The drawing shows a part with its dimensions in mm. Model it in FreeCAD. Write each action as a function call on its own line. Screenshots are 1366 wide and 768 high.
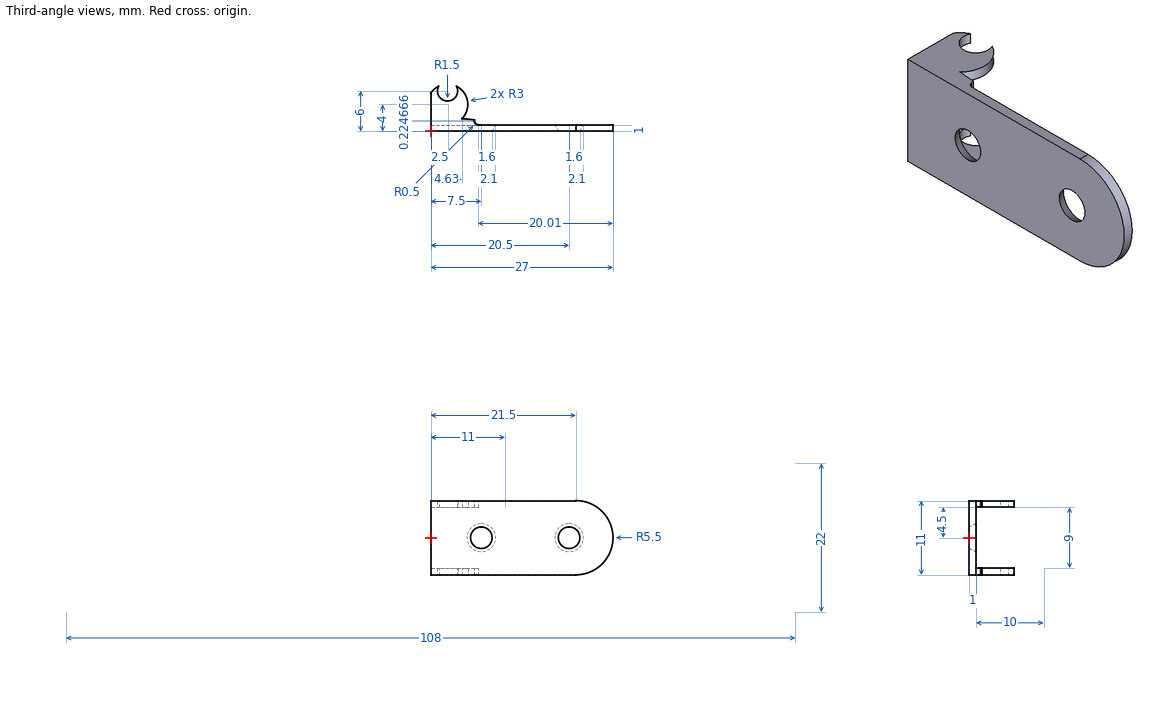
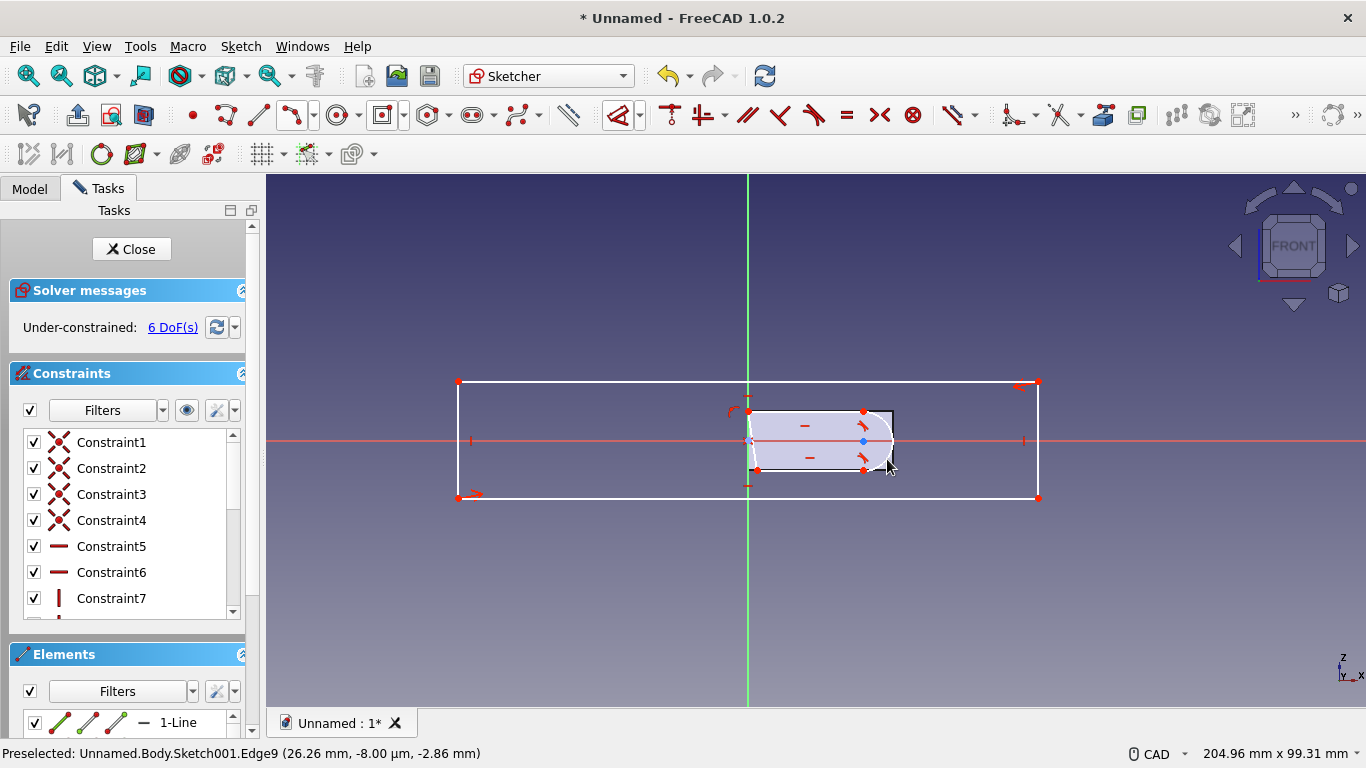
scroll(751, 430, up, 2)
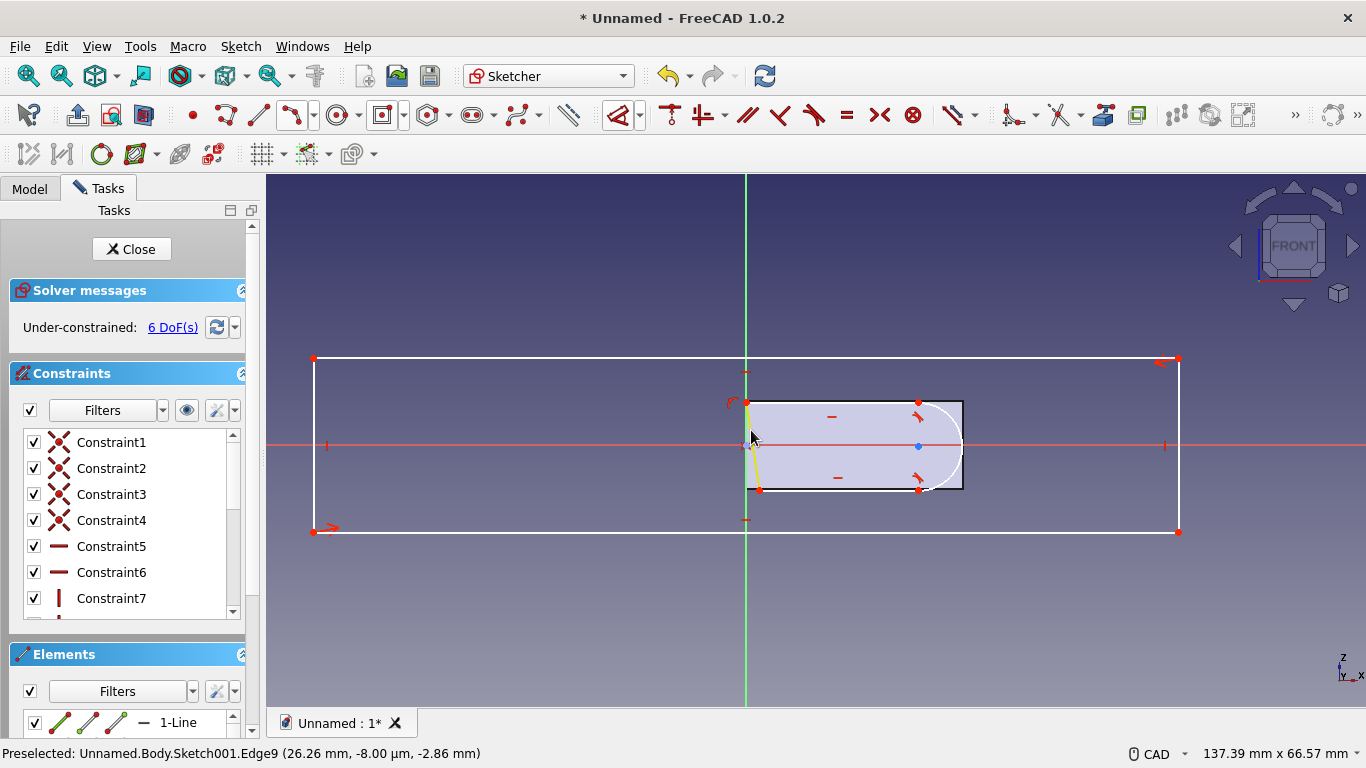
click(750, 429)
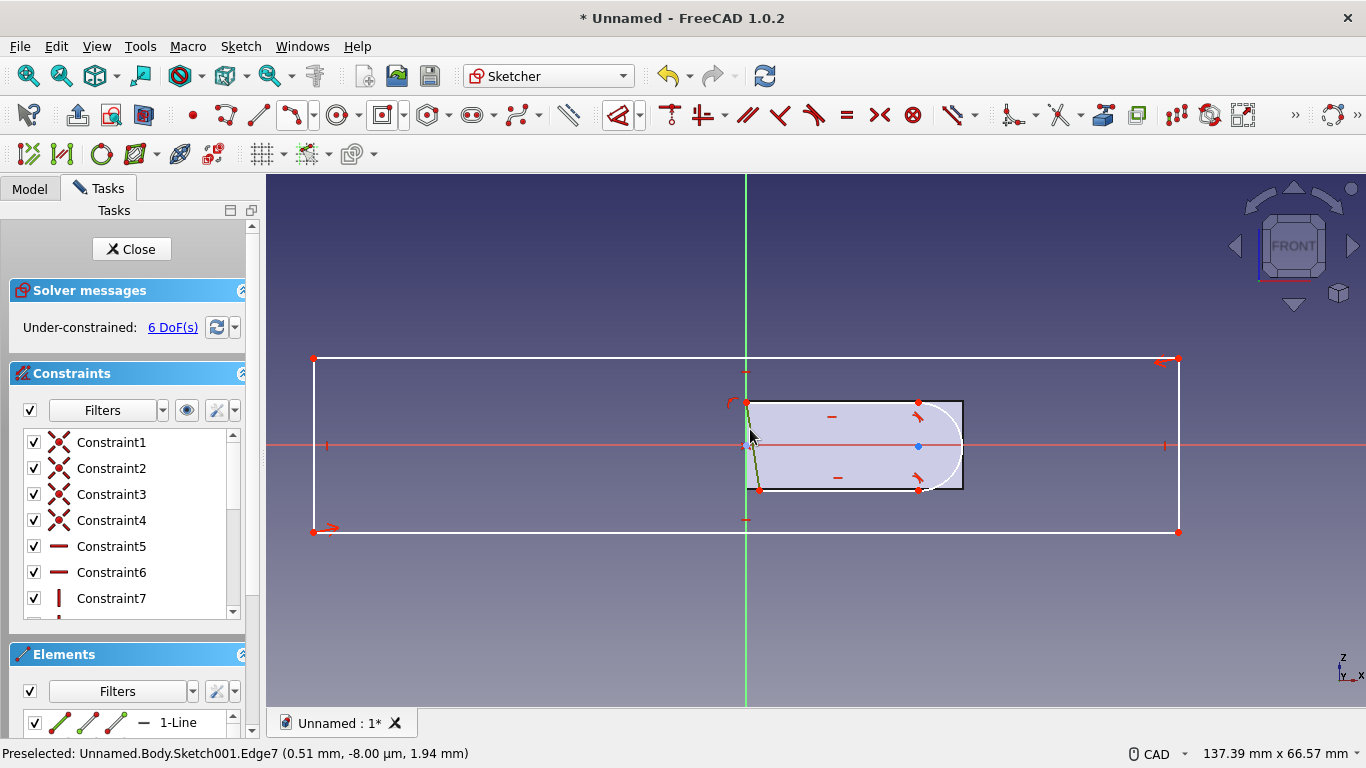
key(v)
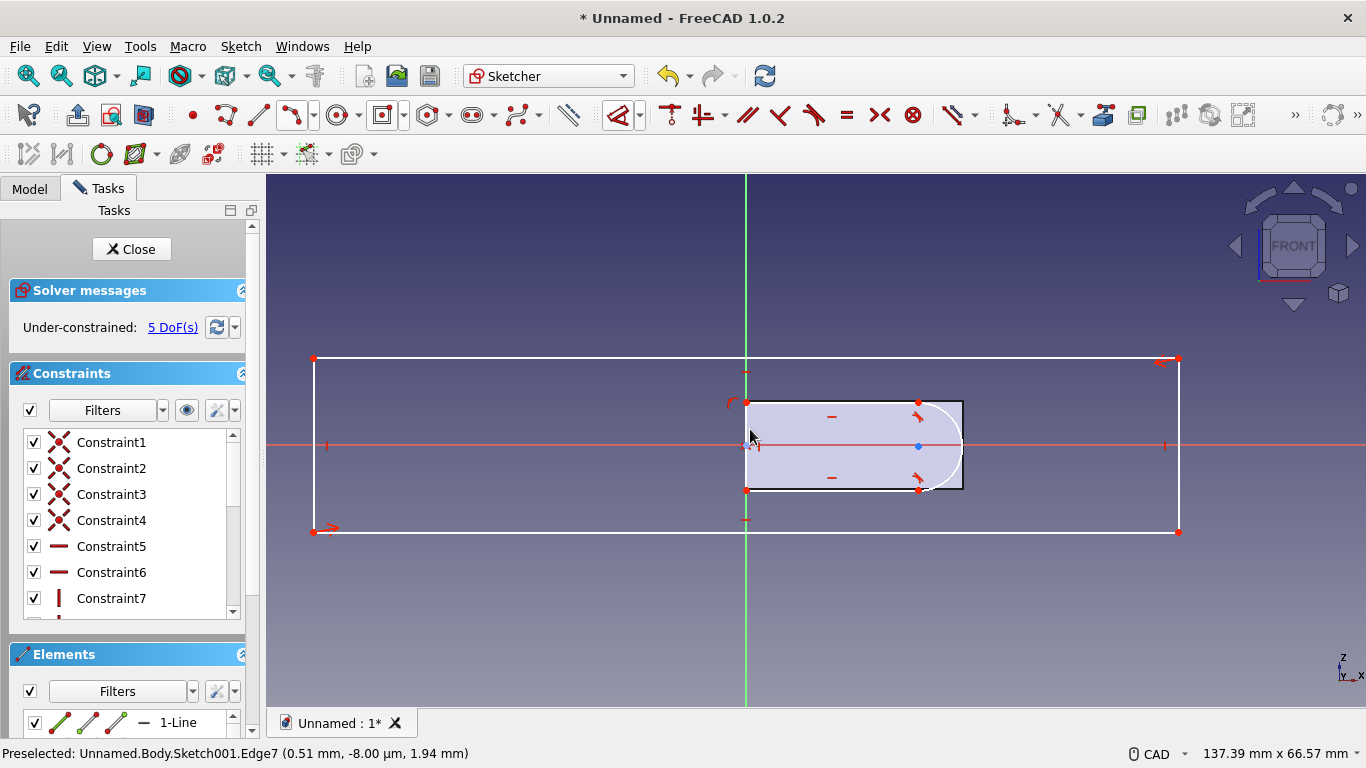
click(918, 447)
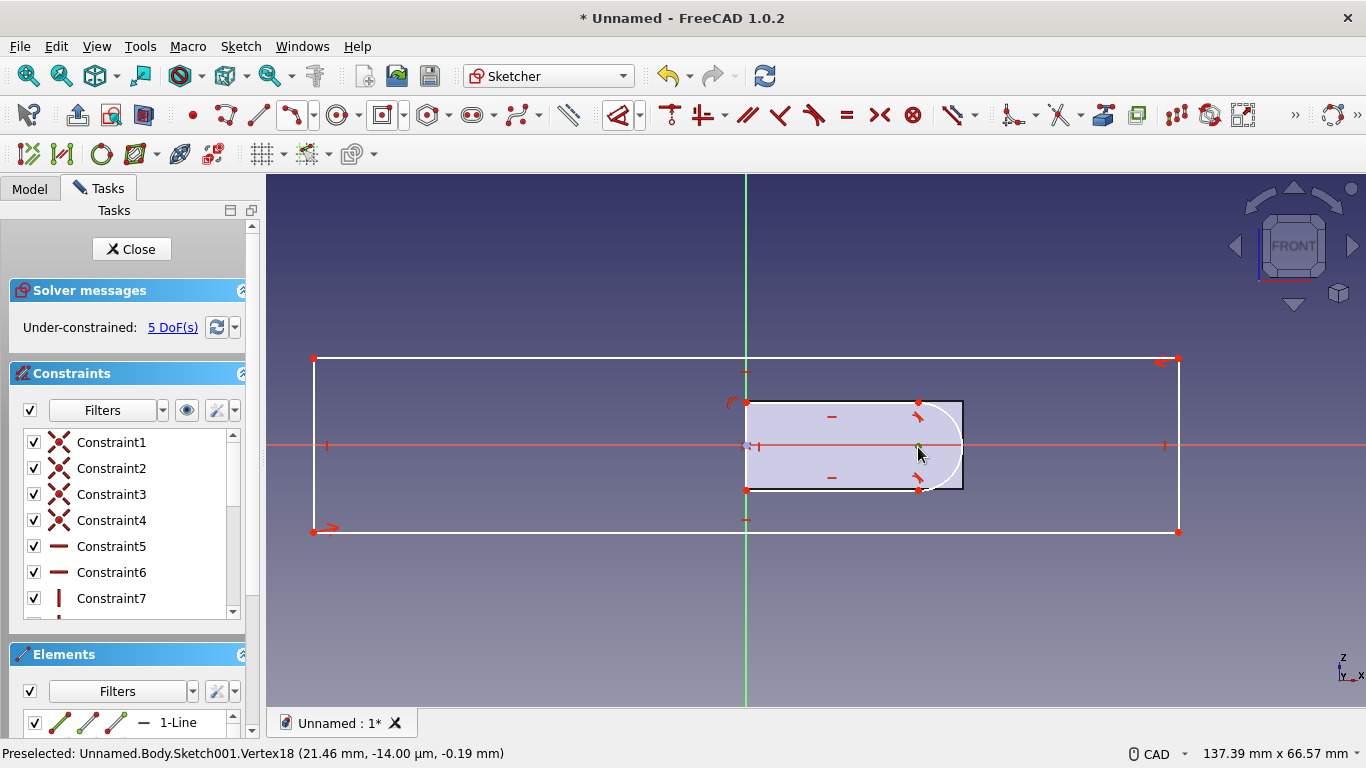
click(359, 445)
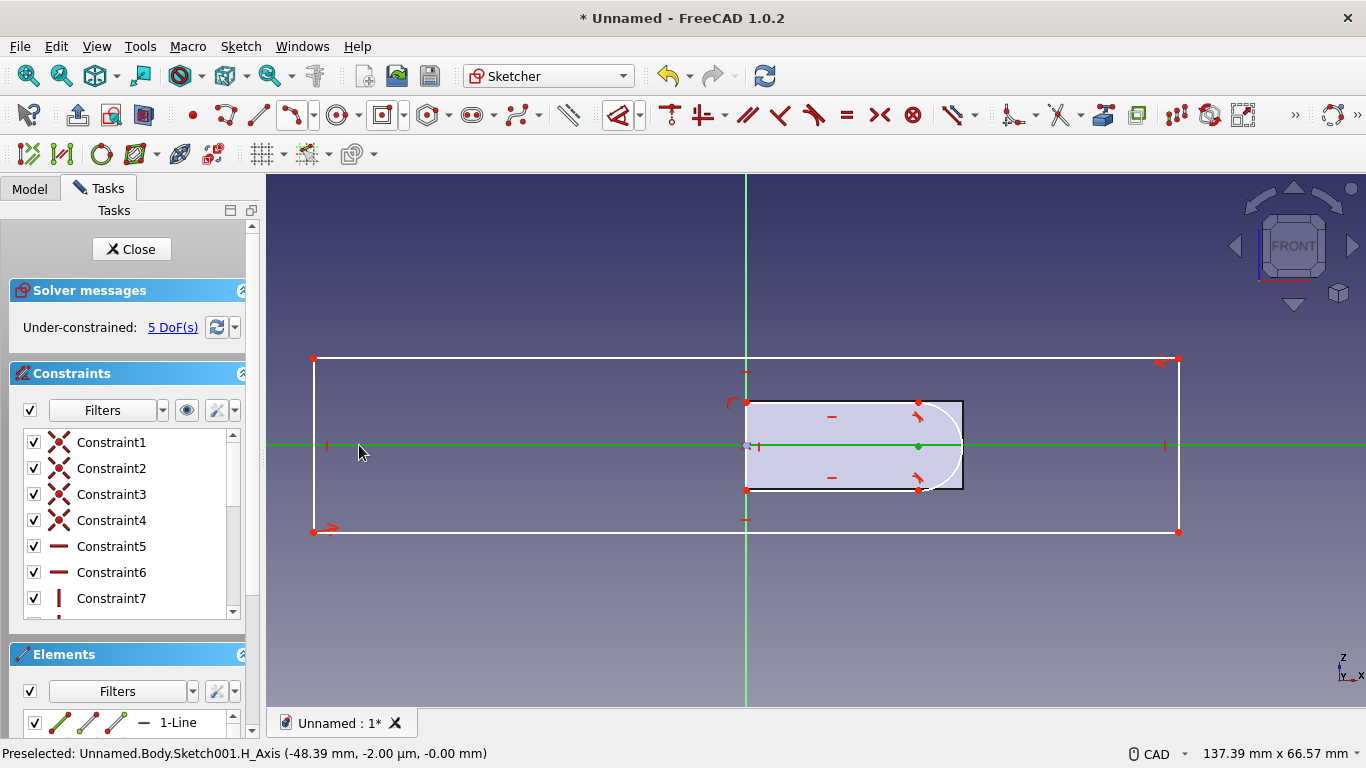
click(670, 116)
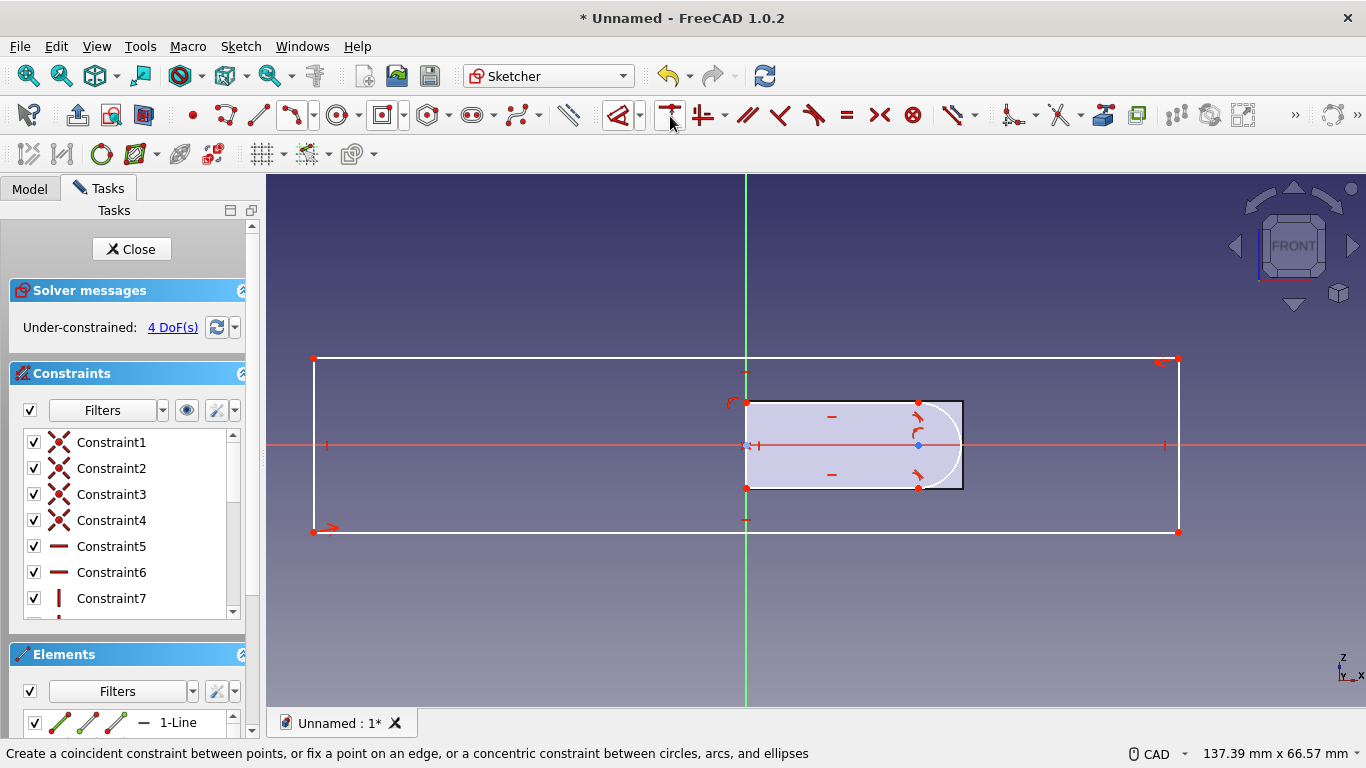
click(953, 470)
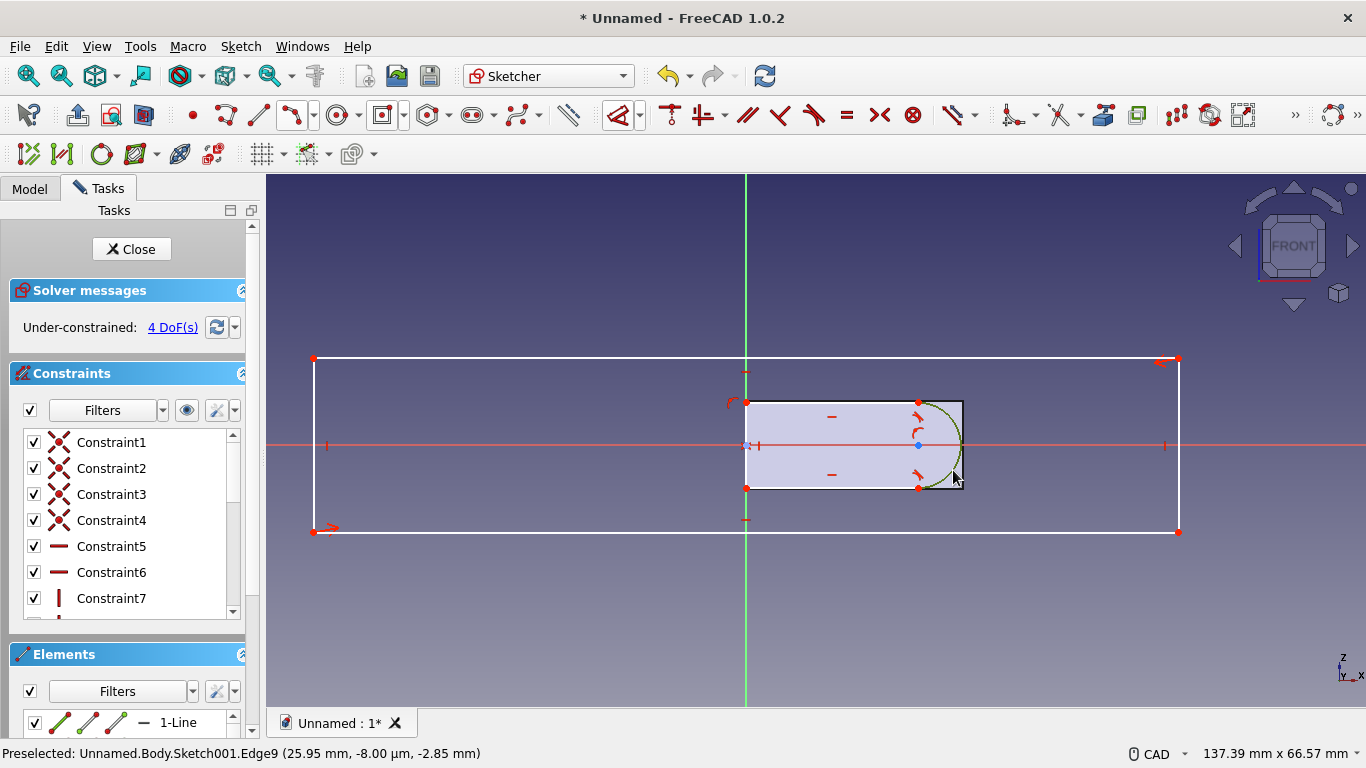
key(k)
key(r)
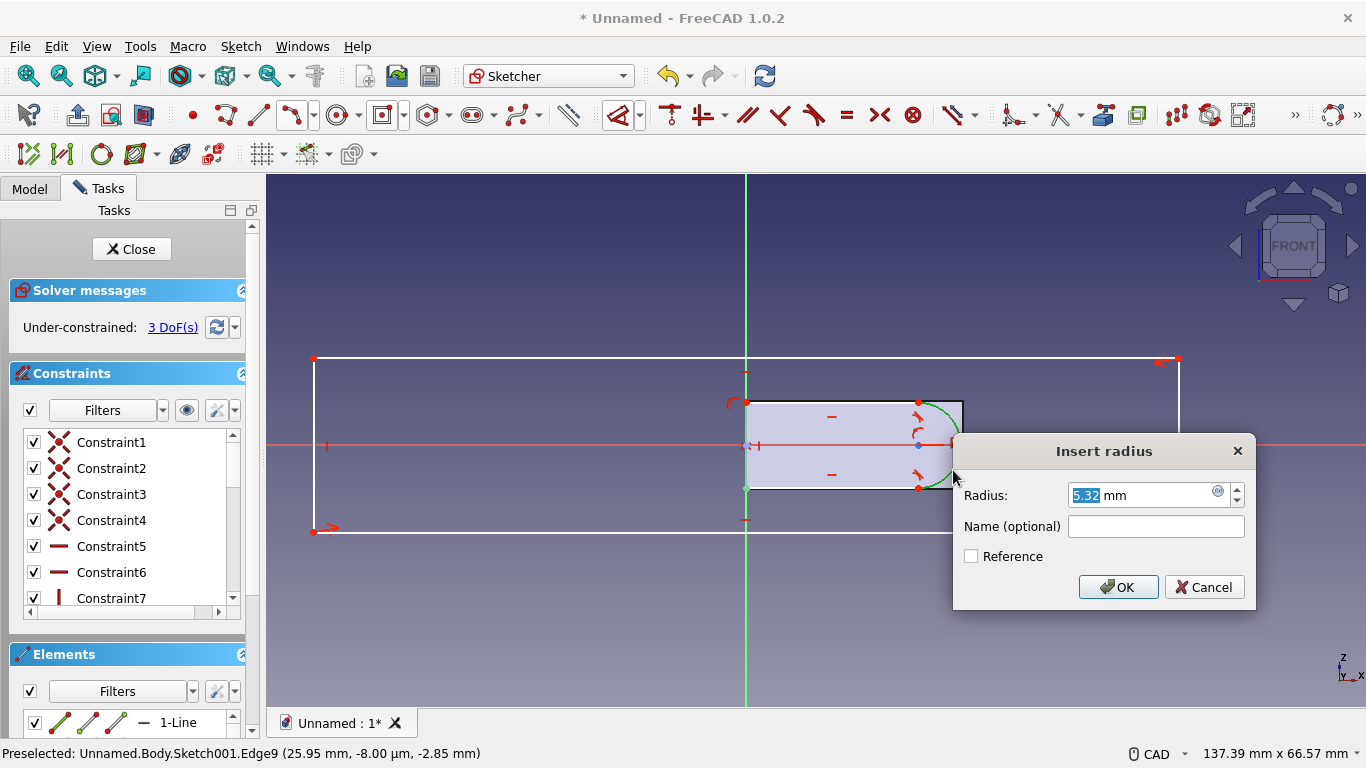
text(5.5)
key(Return)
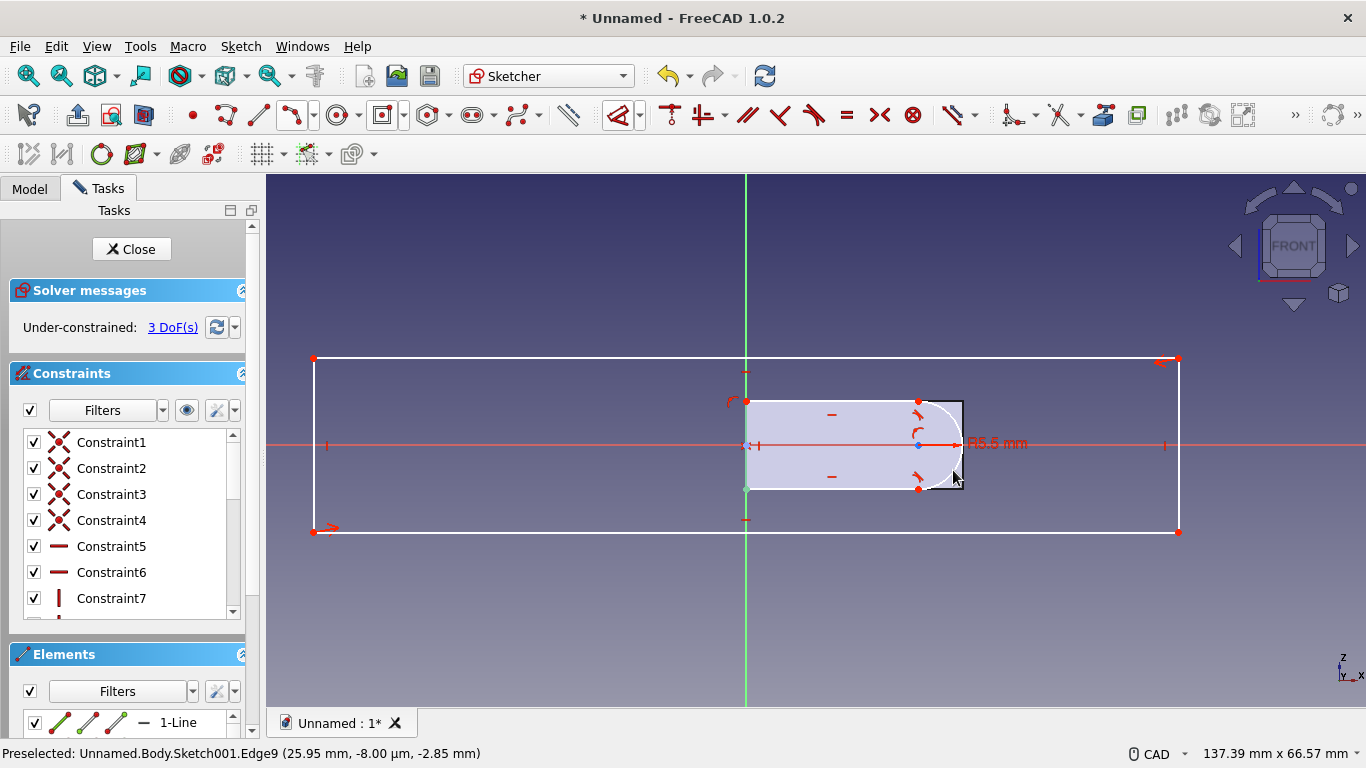
click(1179, 480)